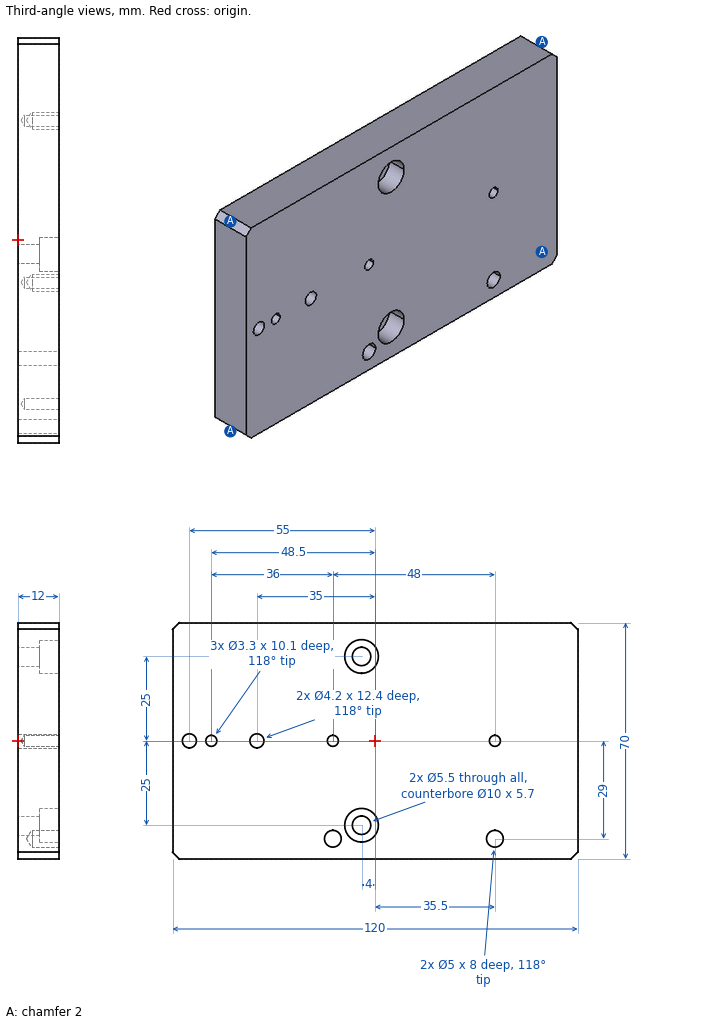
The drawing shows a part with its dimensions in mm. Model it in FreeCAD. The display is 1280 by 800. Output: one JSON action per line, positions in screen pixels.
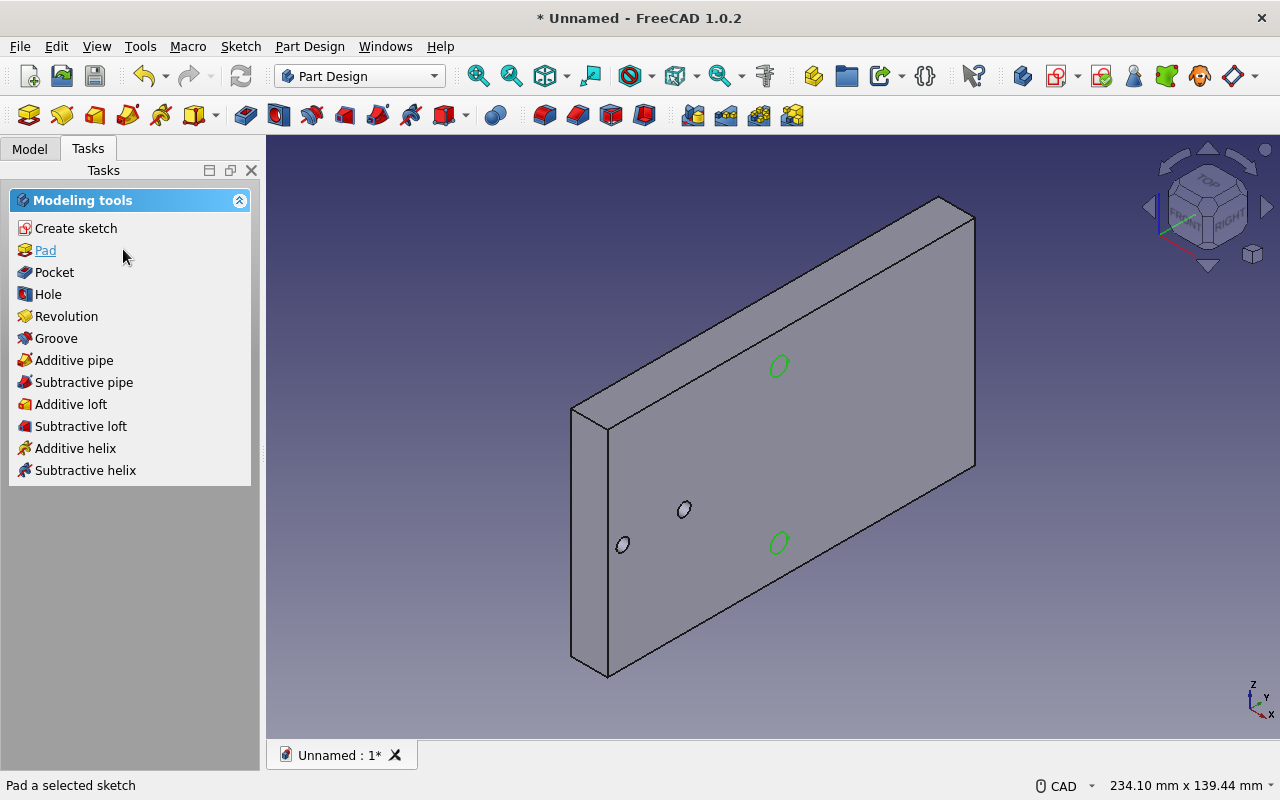
{"action": "left_click", "coordinate": [279, 116]}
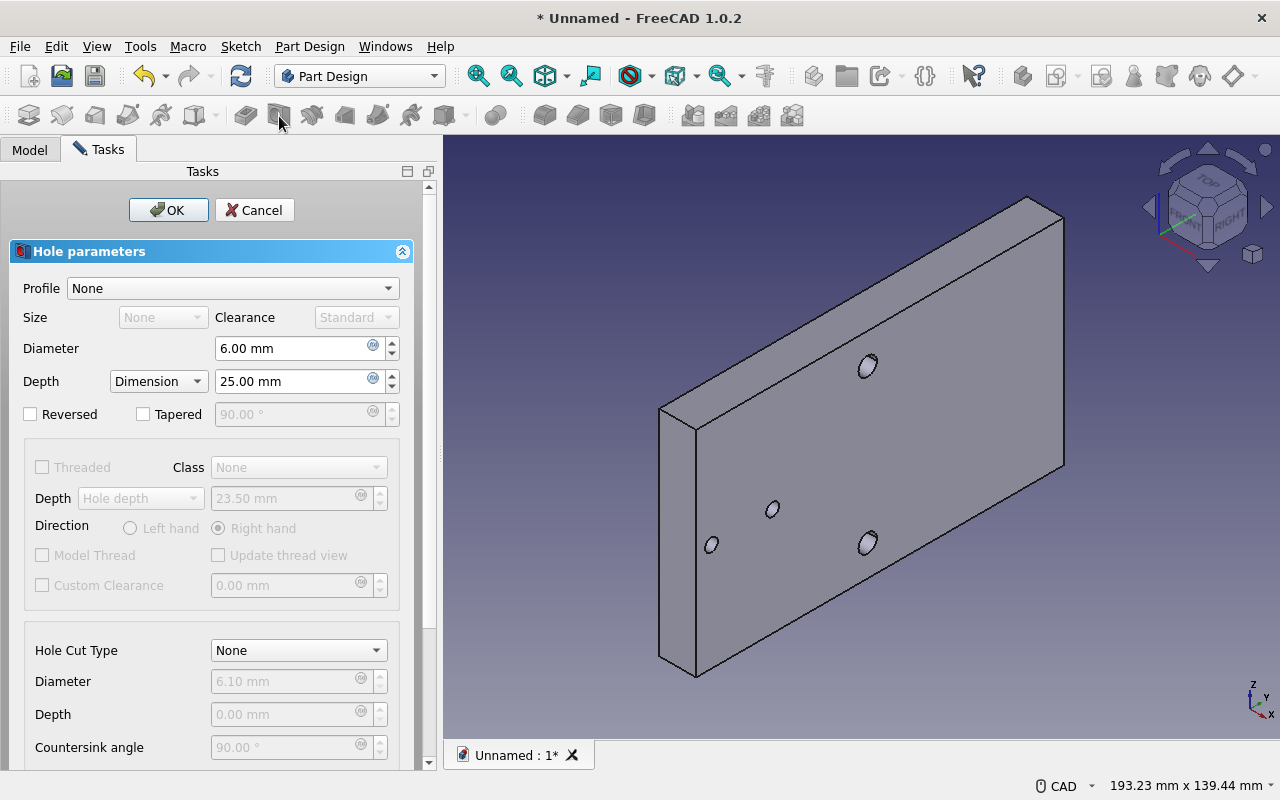
{"action": "triple_click", "coordinate": [300, 348]}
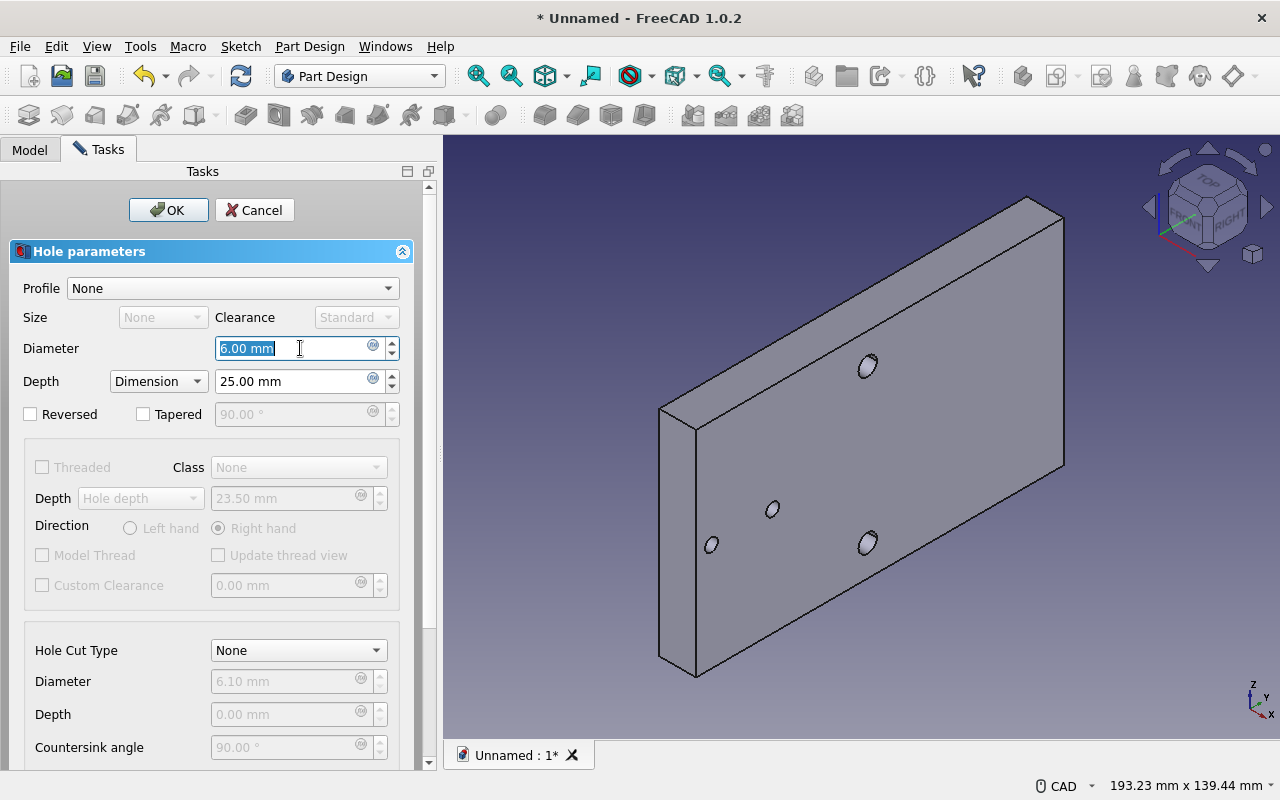
{"action": "type", "text": "5.5"}
{"action": "key", "text": "Tab"}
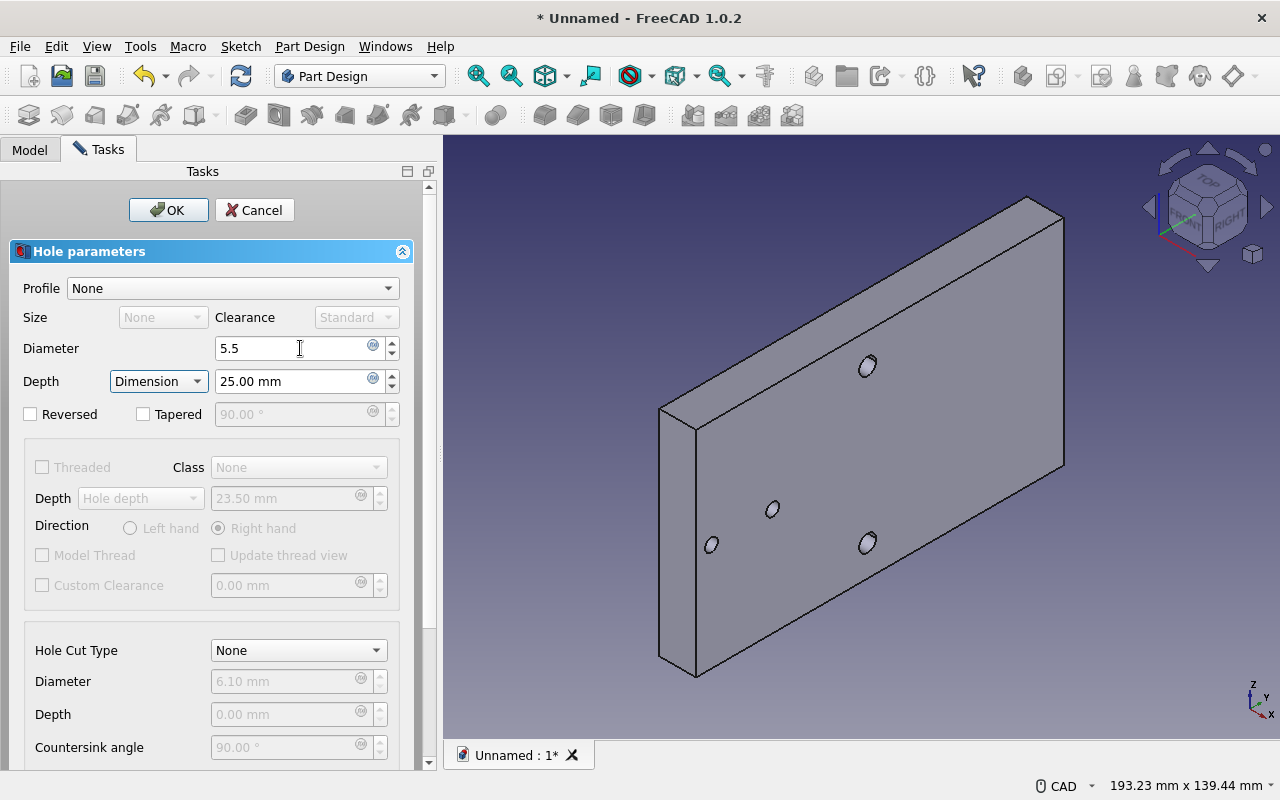
{"action": "left_click", "coordinate": [160, 382]}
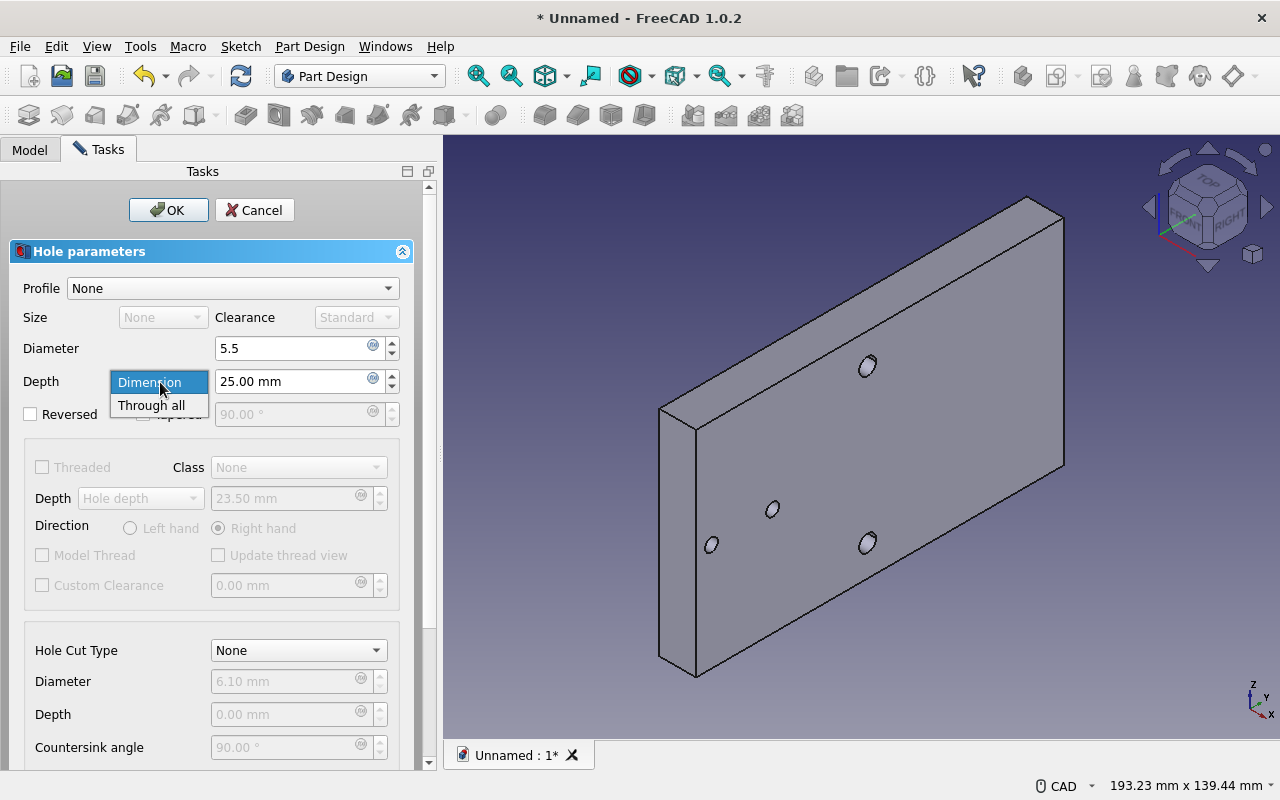
{"action": "left_click", "coordinate": [158, 406]}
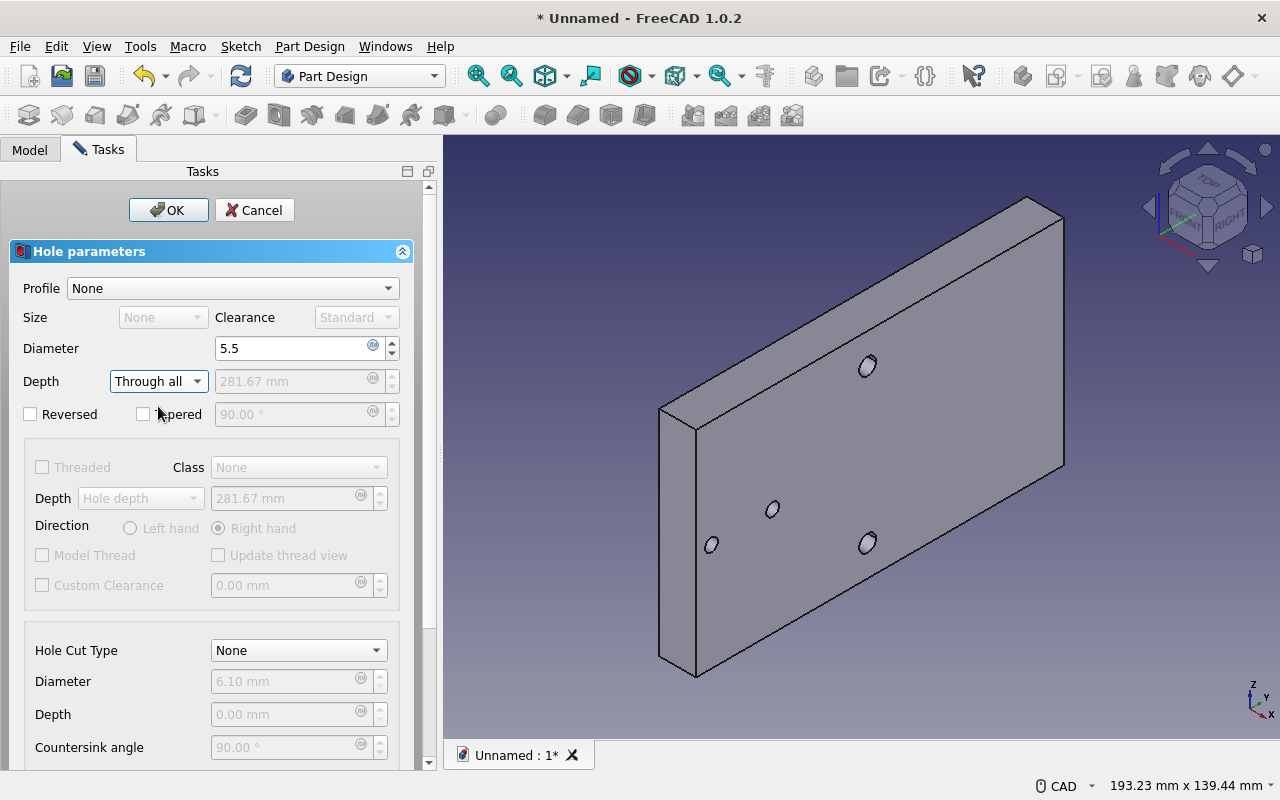
{"action": "left_click", "coordinate": [300, 650]}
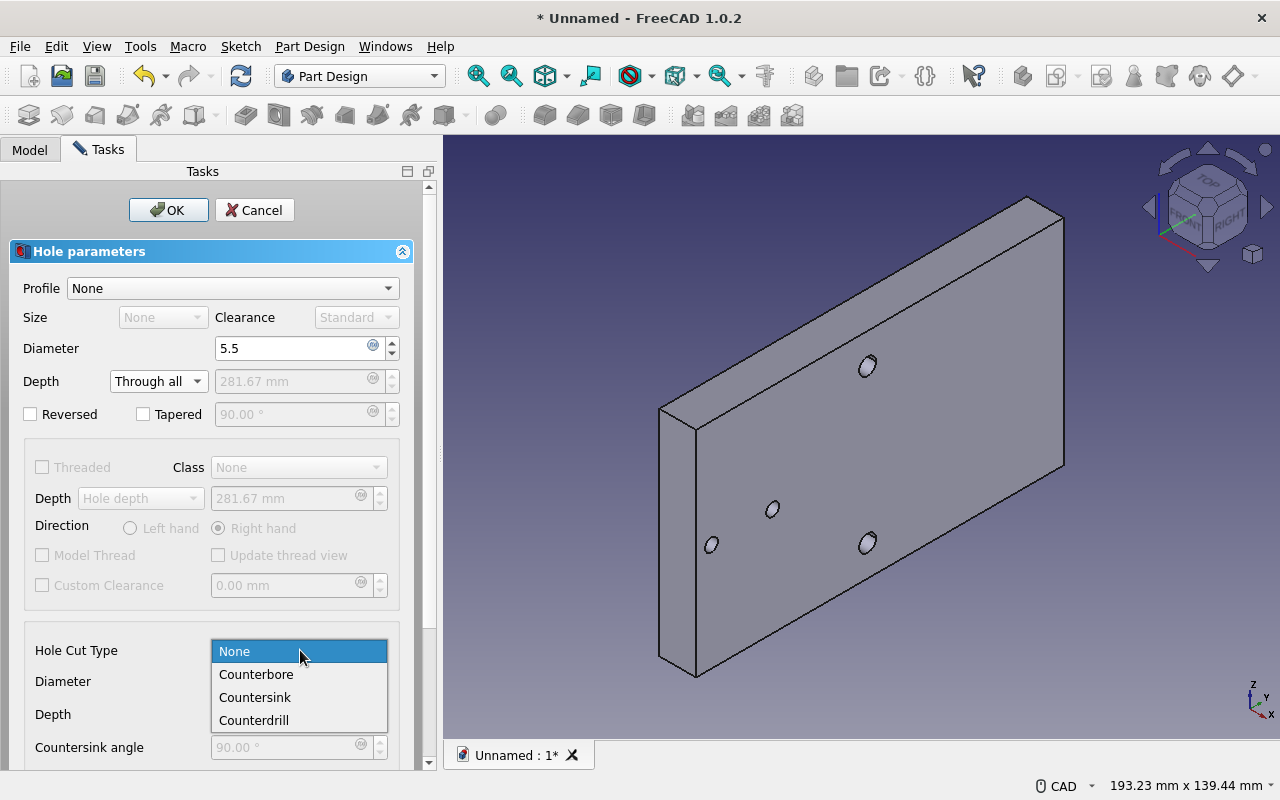
{"action": "left_click", "coordinate": [298, 674]}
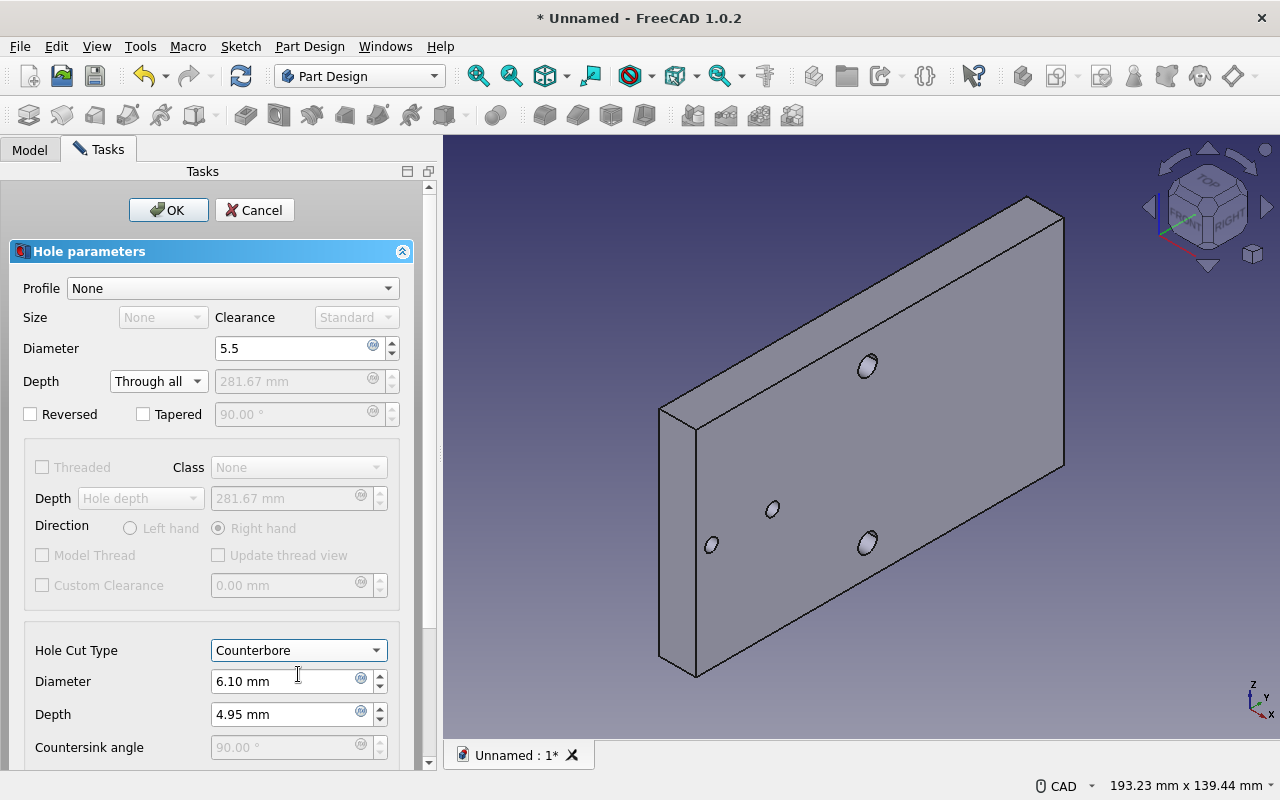
{"action": "triple_click", "coordinate": [292, 682]}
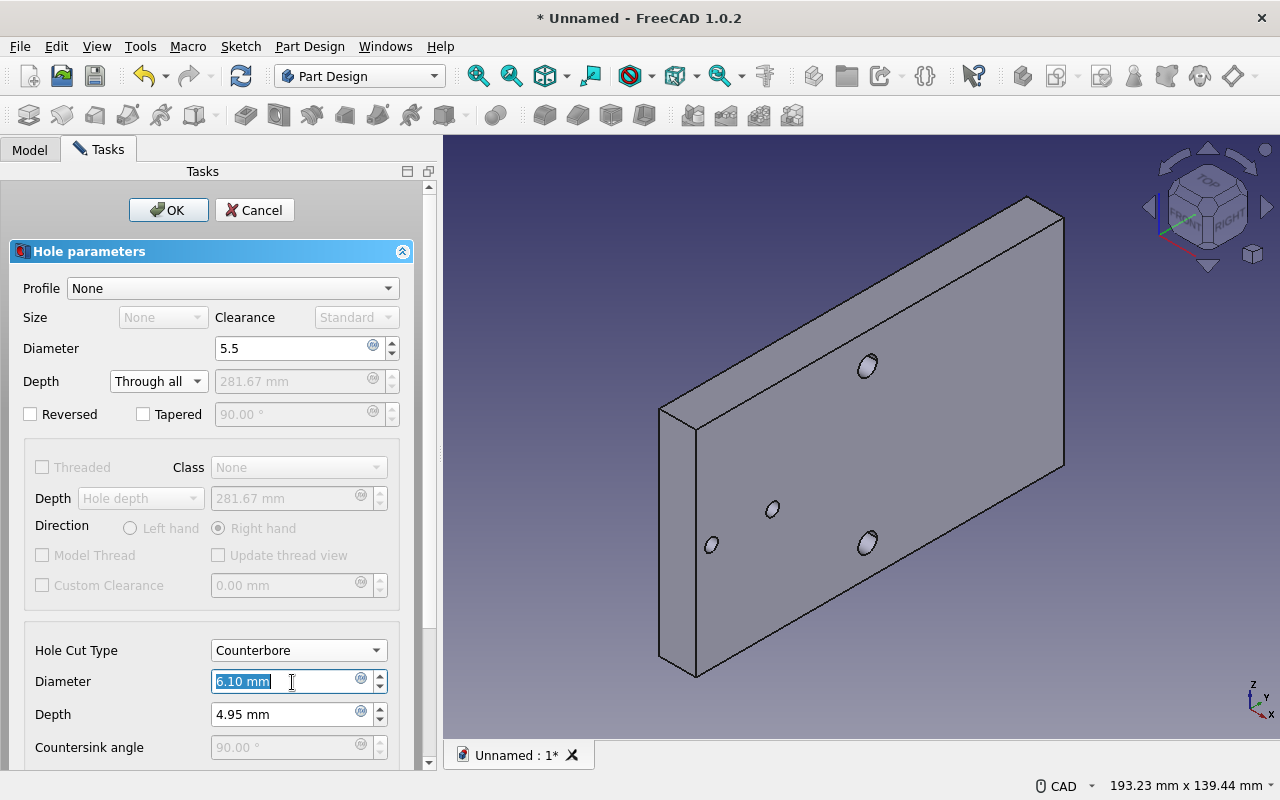
{"action": "type", "text": "10"}
{"action": "key", "text": "Tab"}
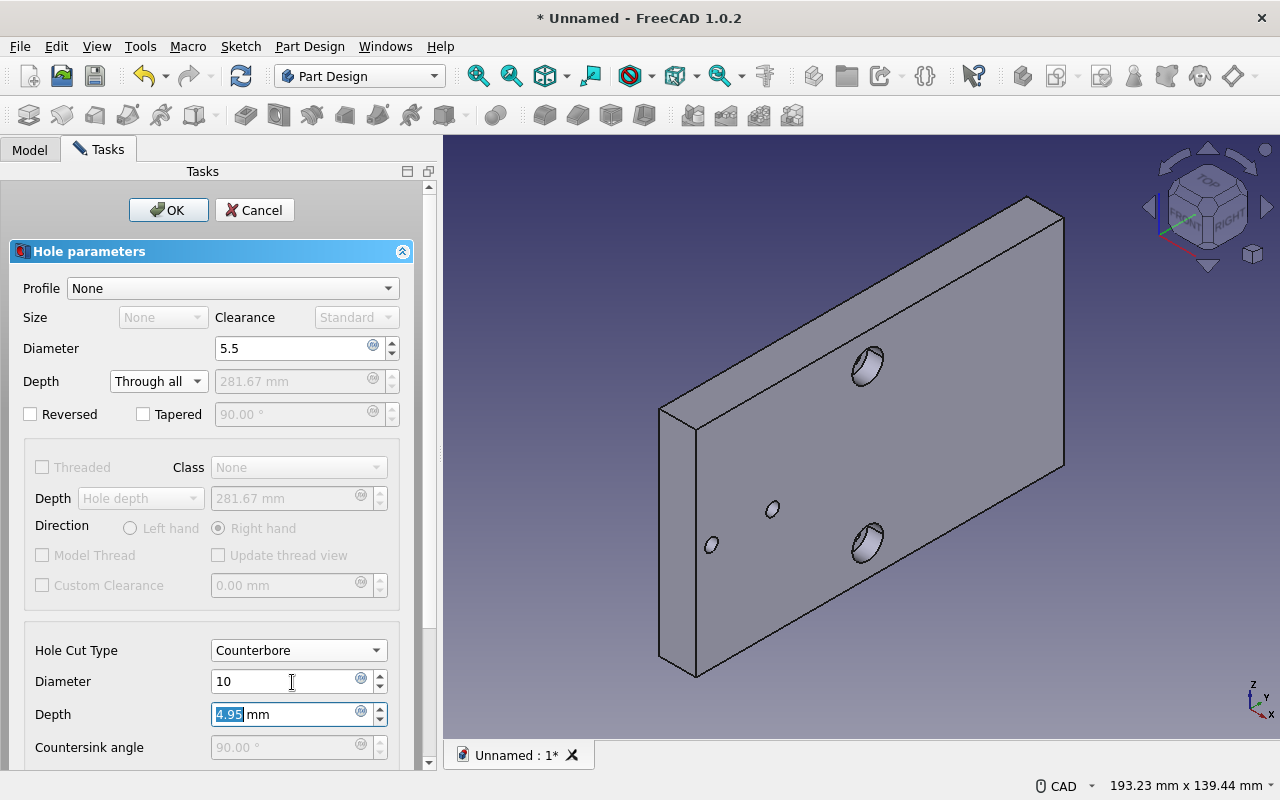
{"action": "type", "text": "5.7"}
{"action": "key", "text": "Tab"}